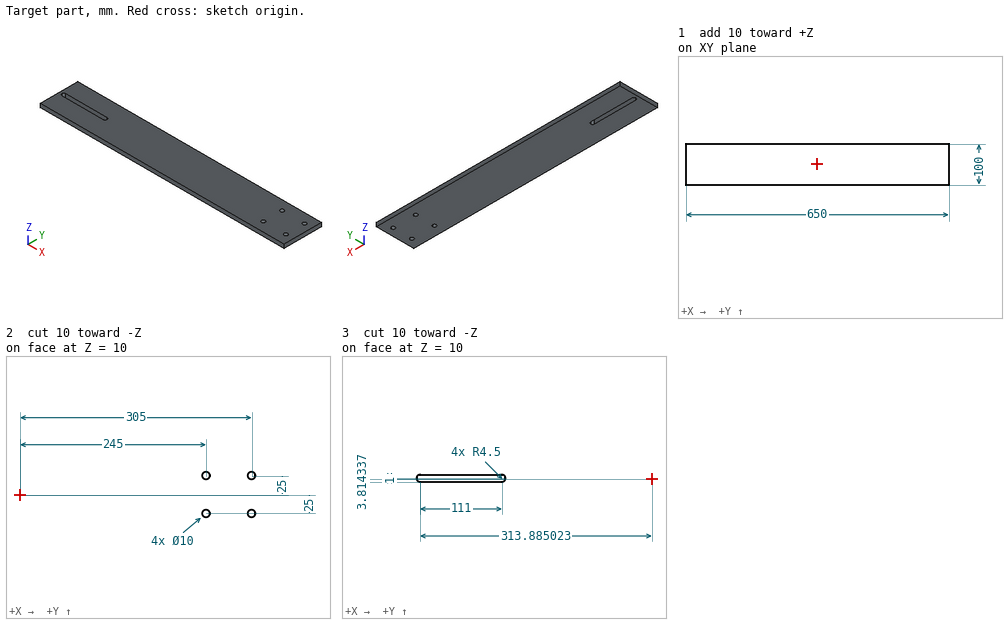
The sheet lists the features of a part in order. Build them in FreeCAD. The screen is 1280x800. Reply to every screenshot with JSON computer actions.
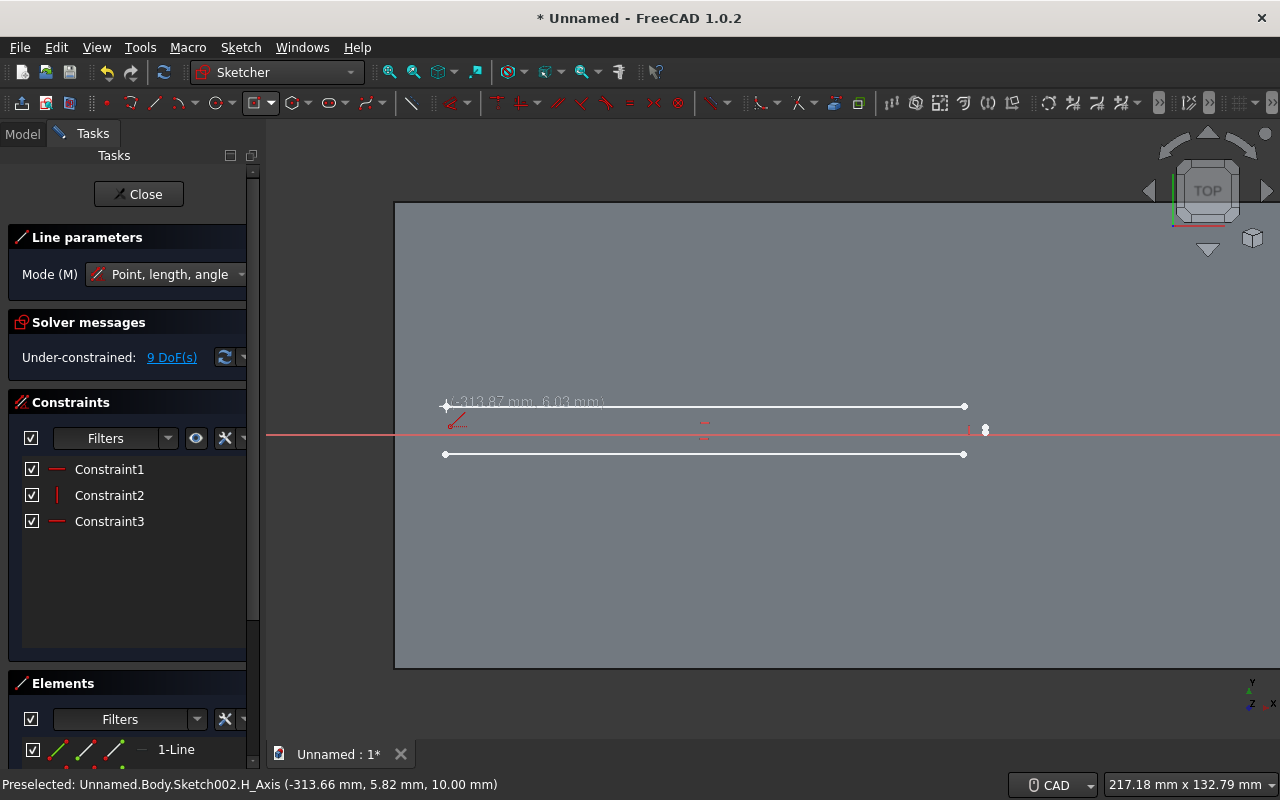
{"action": "scroll", "coordinate": [425, 427], "scroll_direction": "up", "scroll_amount": 4}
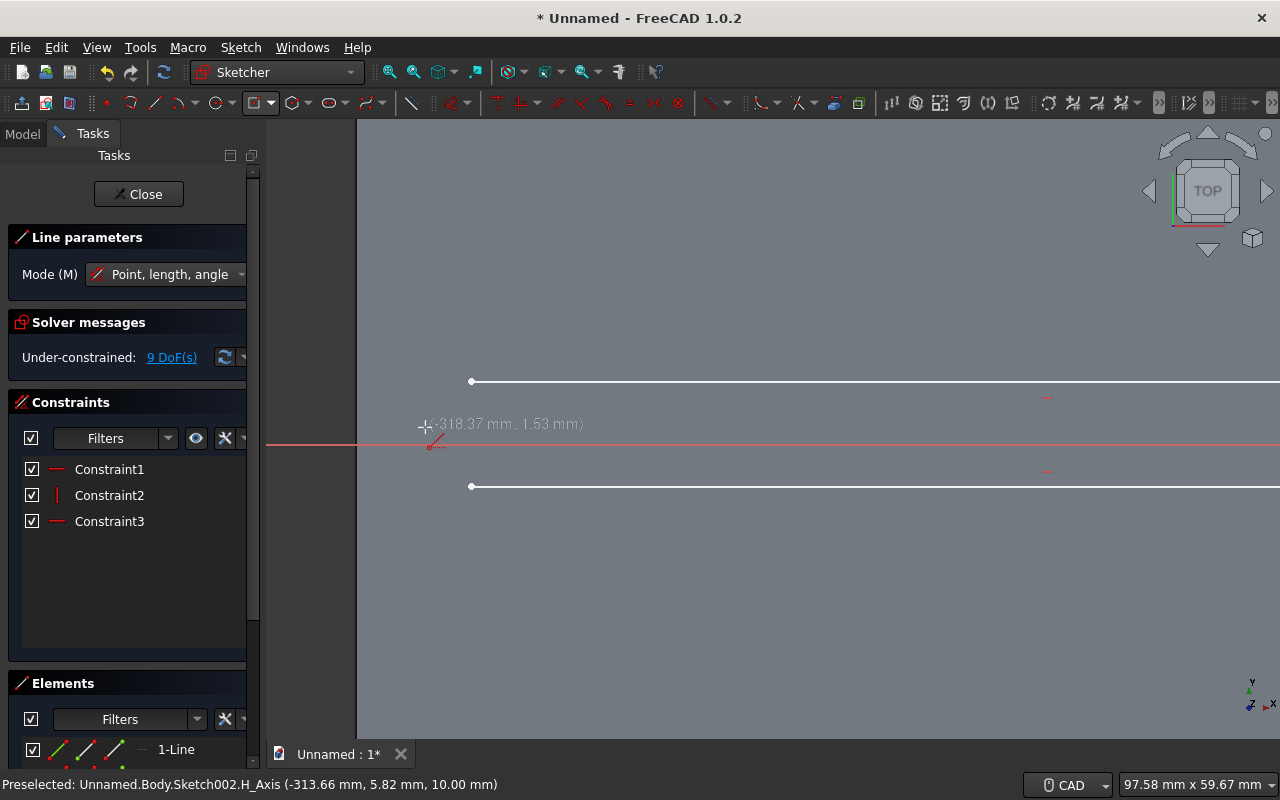
{"action": "left_click", "coordinate": [425, 427]}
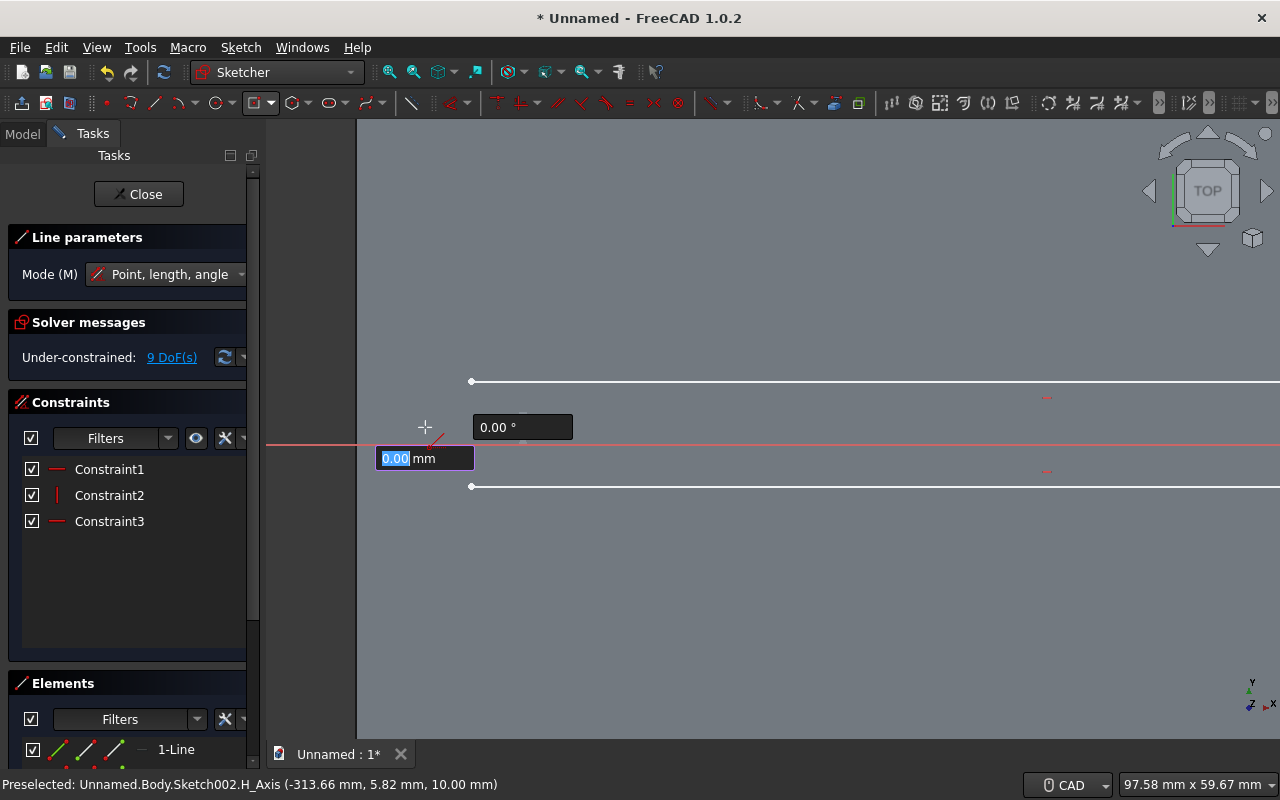
{"action": "scroll", "coordinate": [425, 437], "scroll_direction": "up", "scroll_amount": 5}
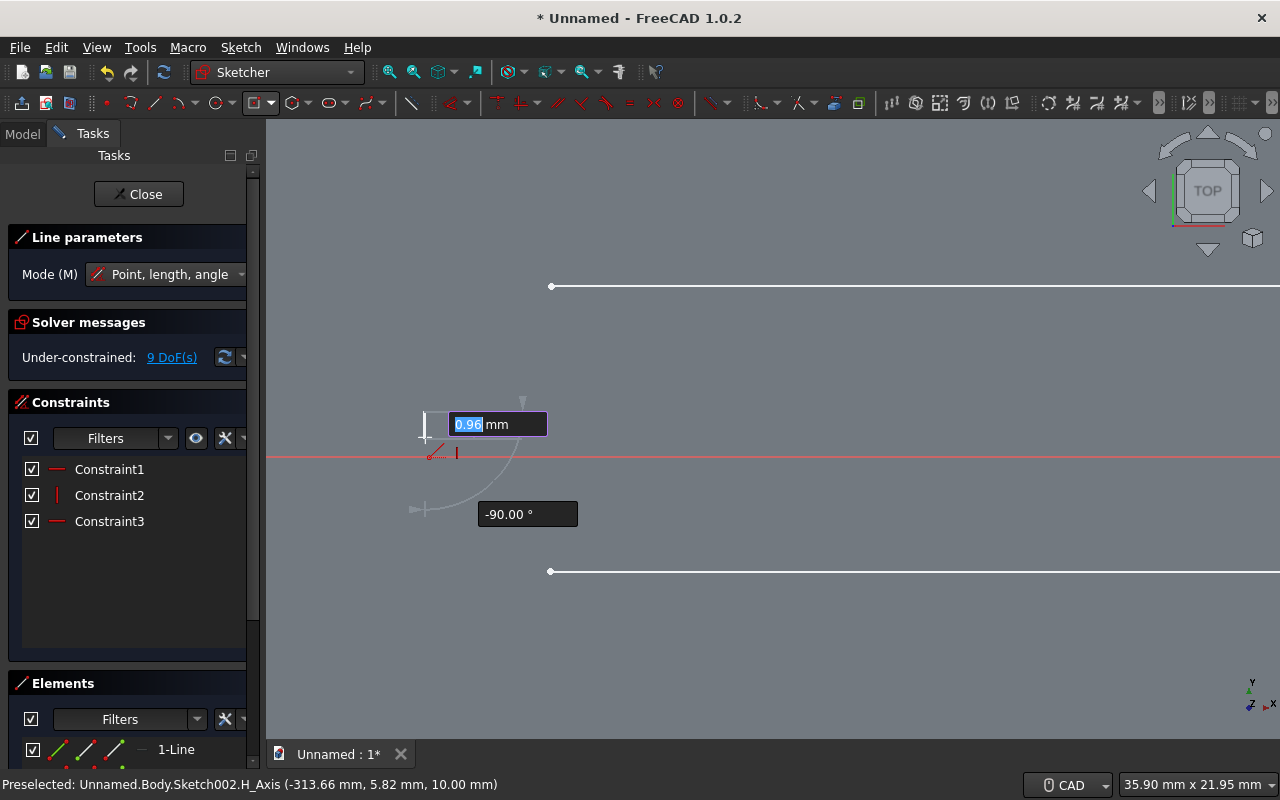
{"action": "left_click", "coordinate": [425, 437]}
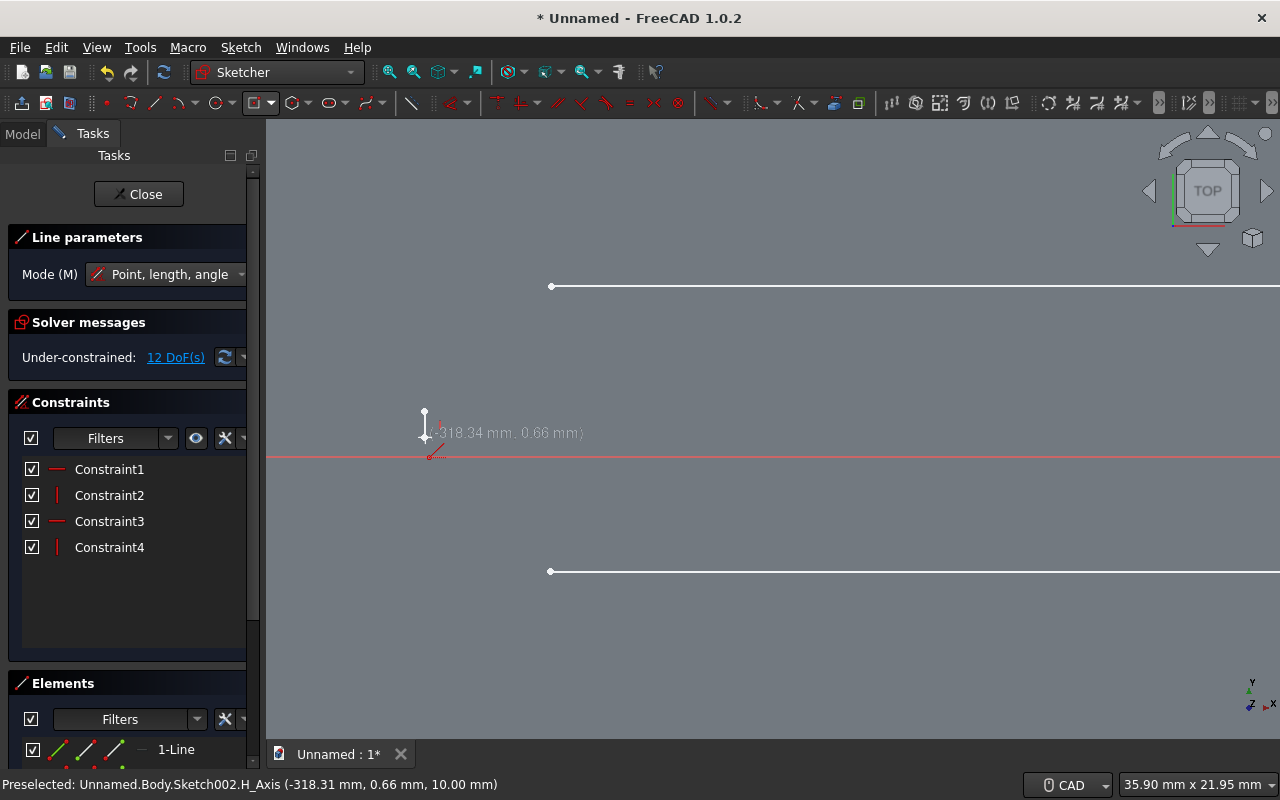
{"action": "key", "text": "g 3 a"}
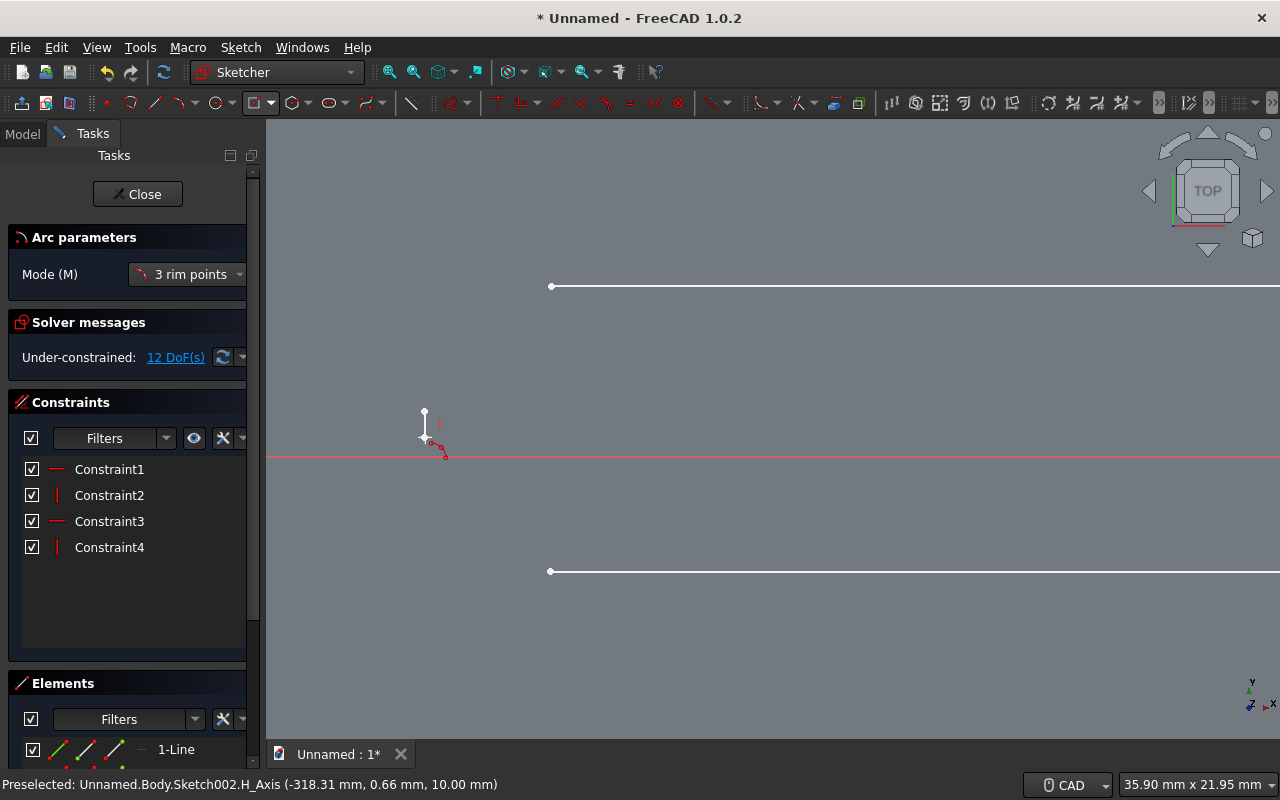
{"action": "scroll", "coordinate": [424, 430], "scroll_direction": "down", "scroll_amount": 9}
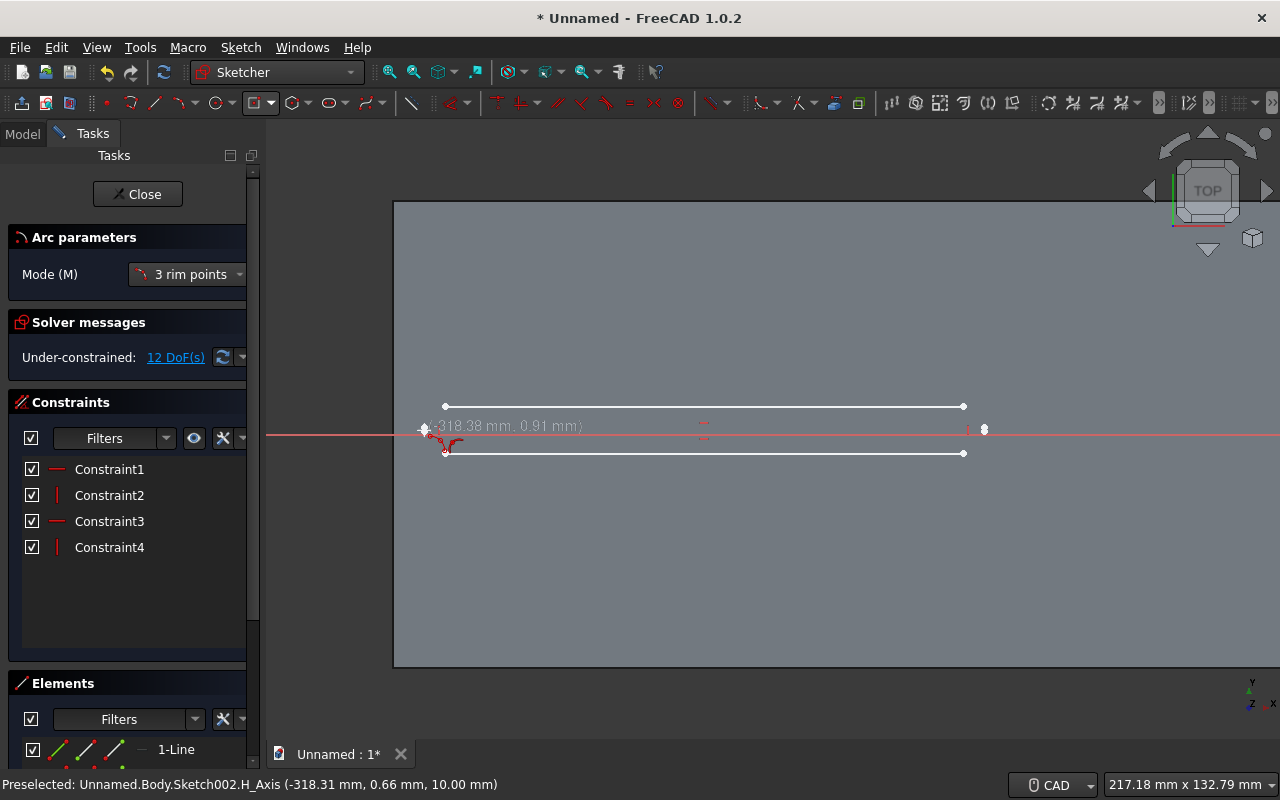
{"action": "left_click", "coordinate": [963, 454]}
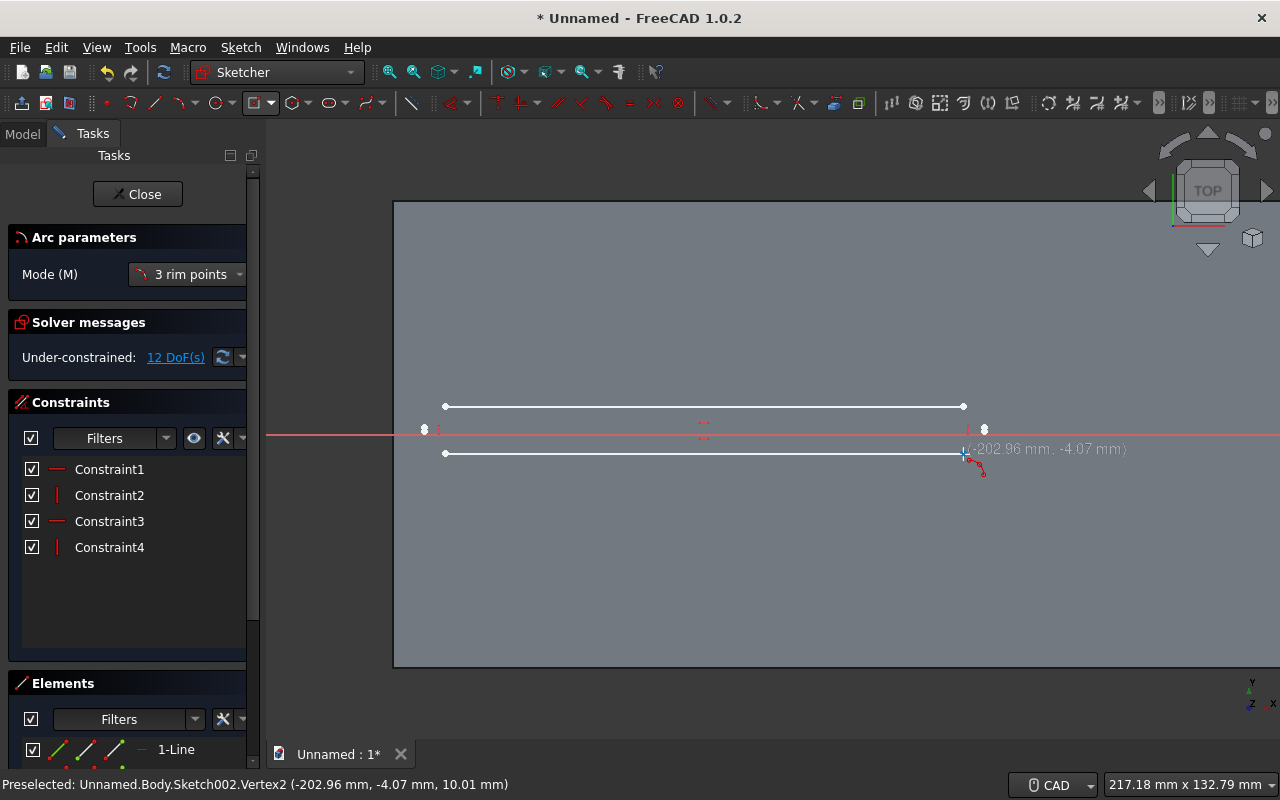
{"action": "scroll", "coordinate": [984, 432], "scroll_direction": "up", "scroll_amount": 10}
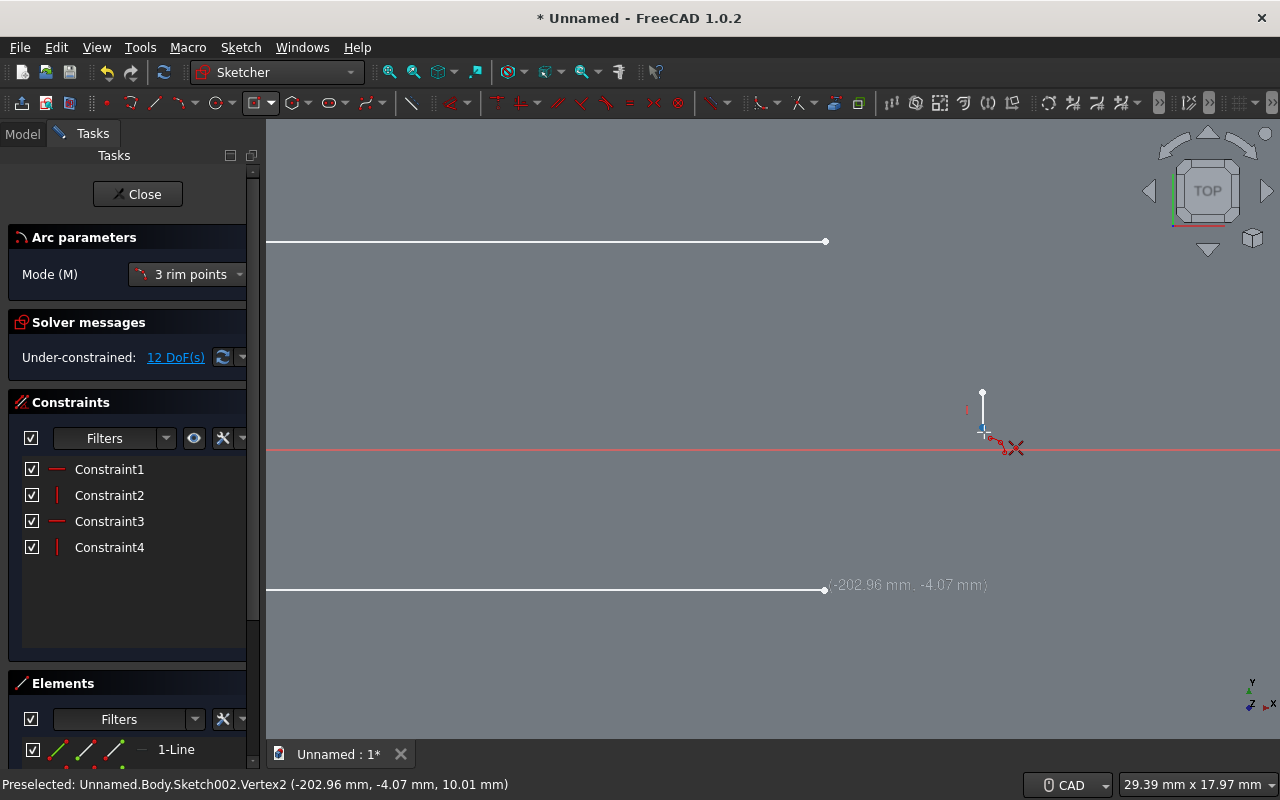
{"action": "left_click", "coordinate": [983, 427]}
{"action": "left_click", "coordinate": [937, 536]}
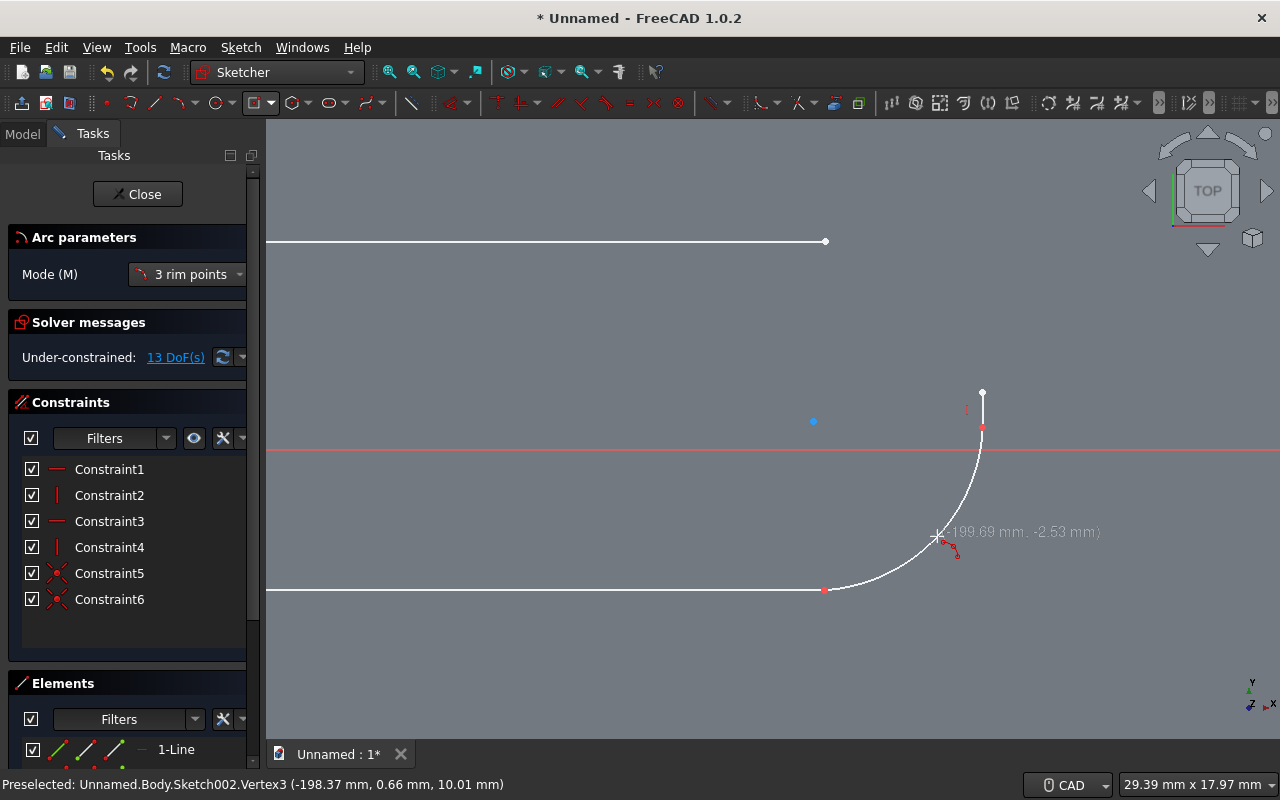
{"action": "left_click", "coordinate": [983, 393]}